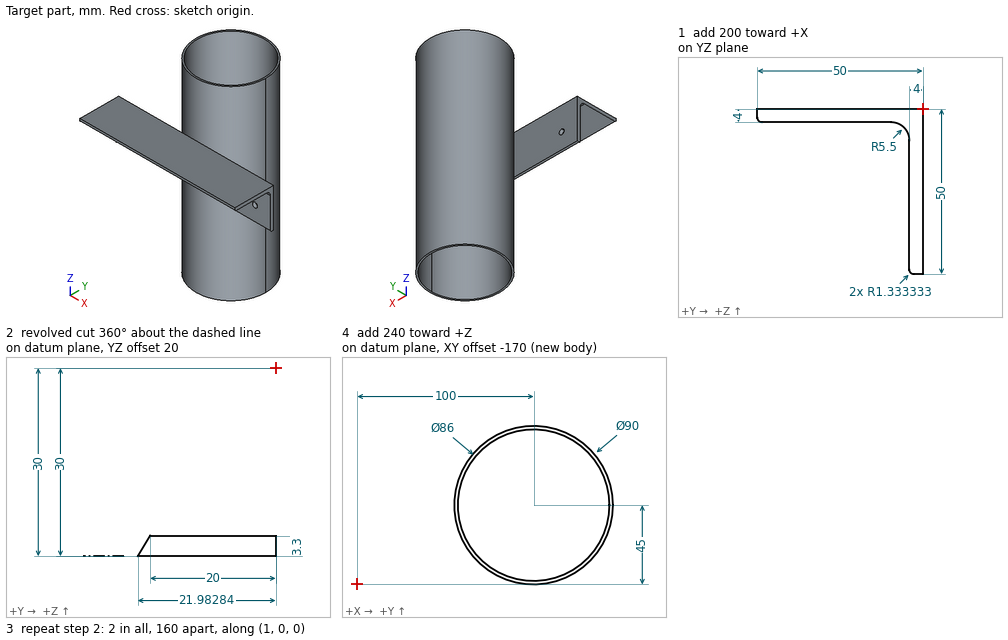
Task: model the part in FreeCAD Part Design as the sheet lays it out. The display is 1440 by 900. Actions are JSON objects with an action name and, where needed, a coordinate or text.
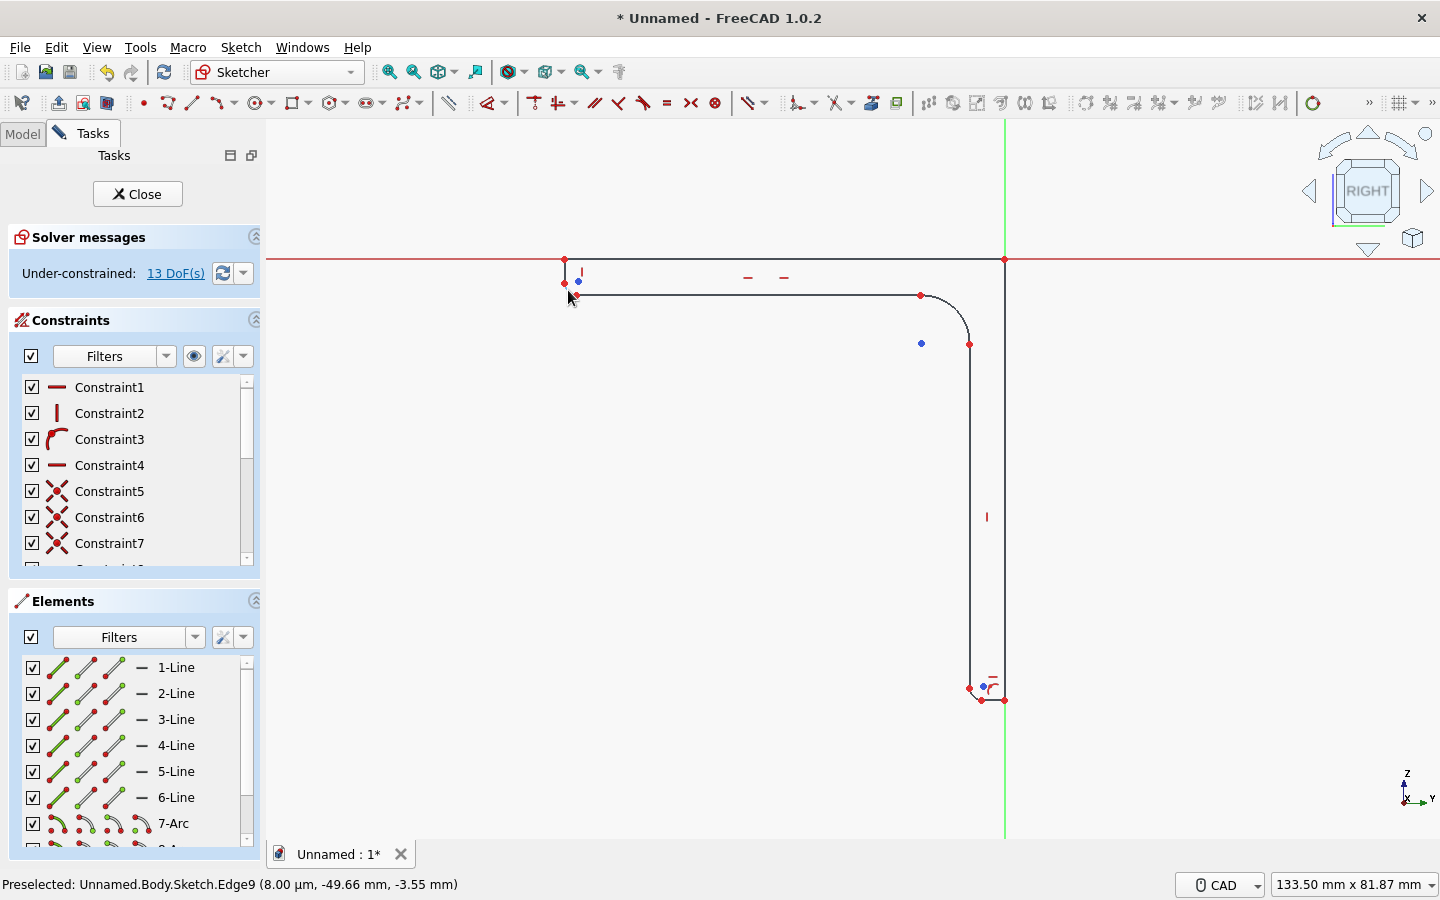
{"action": "left_click", "coordinate": [680, 295]}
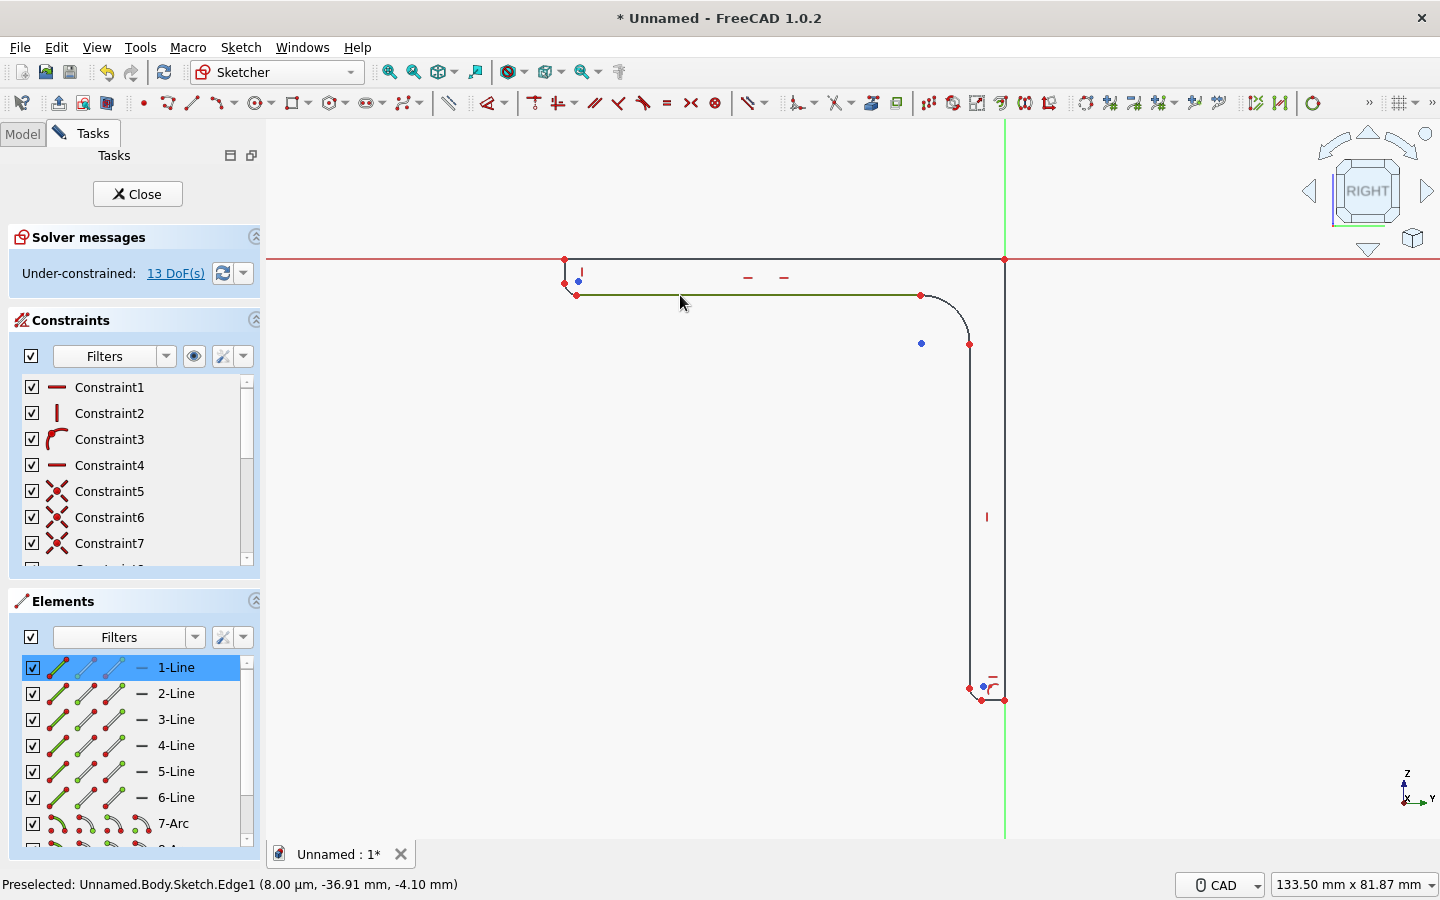
{"action": "left_click", "coordinate": [965, 322]}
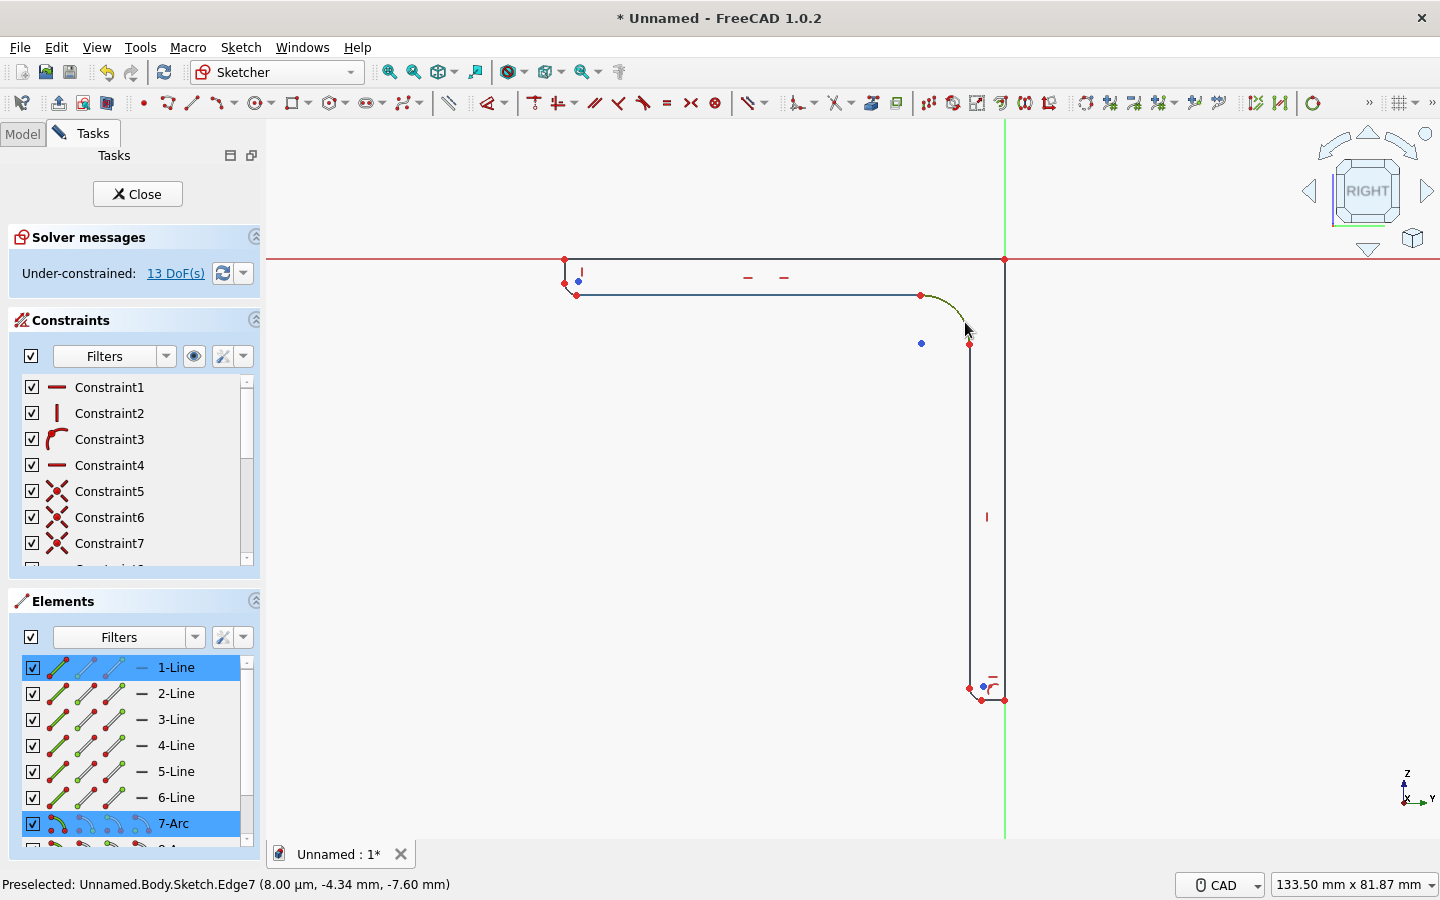
{"action": "left_click", "coordinate": [644, 104]}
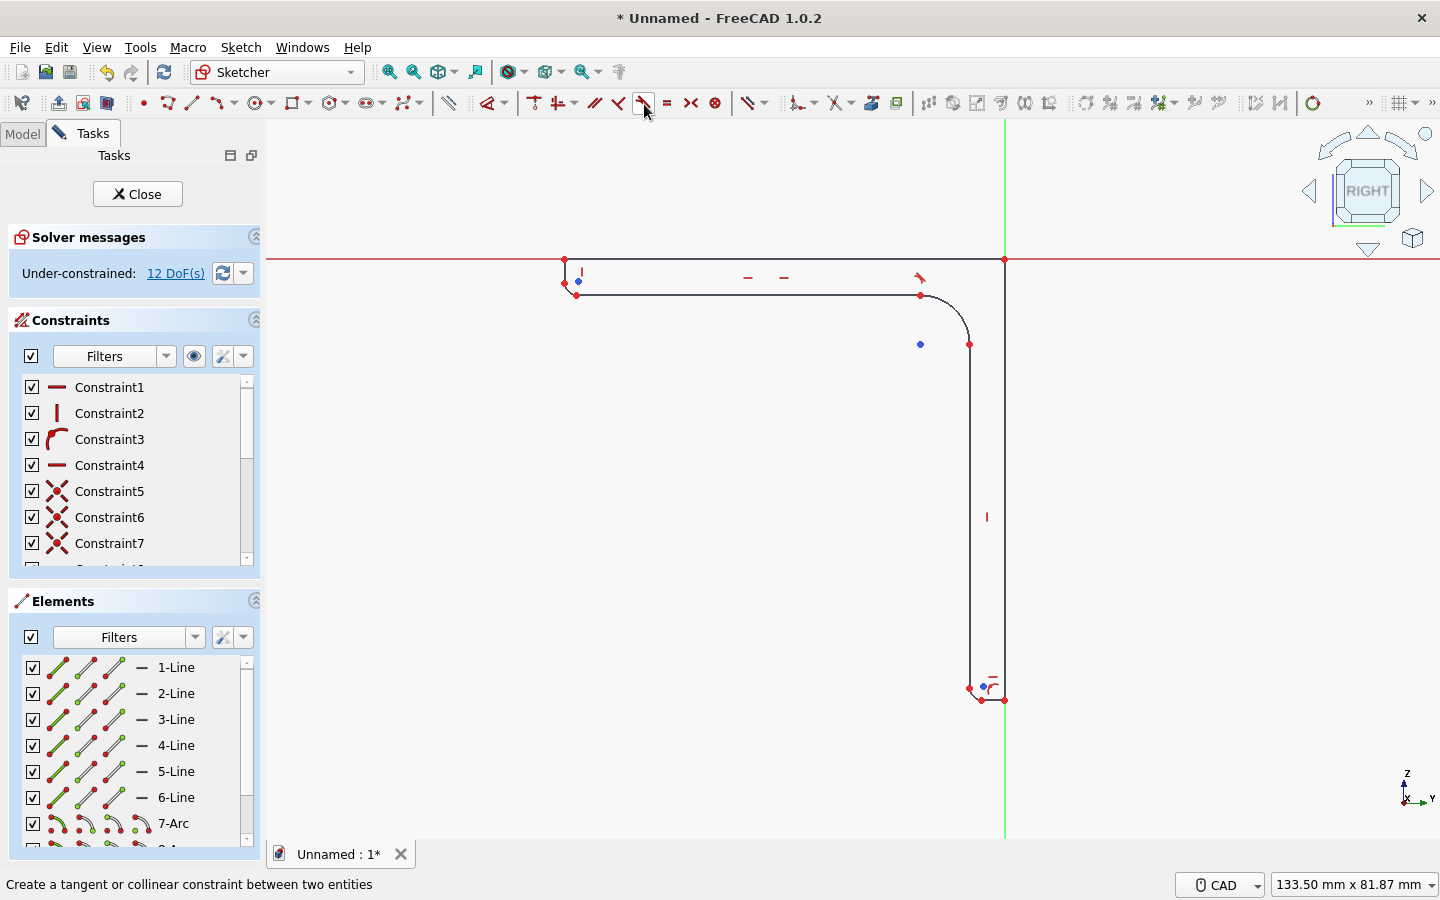
{"action": "left_click", "coordinate": [680, 295]}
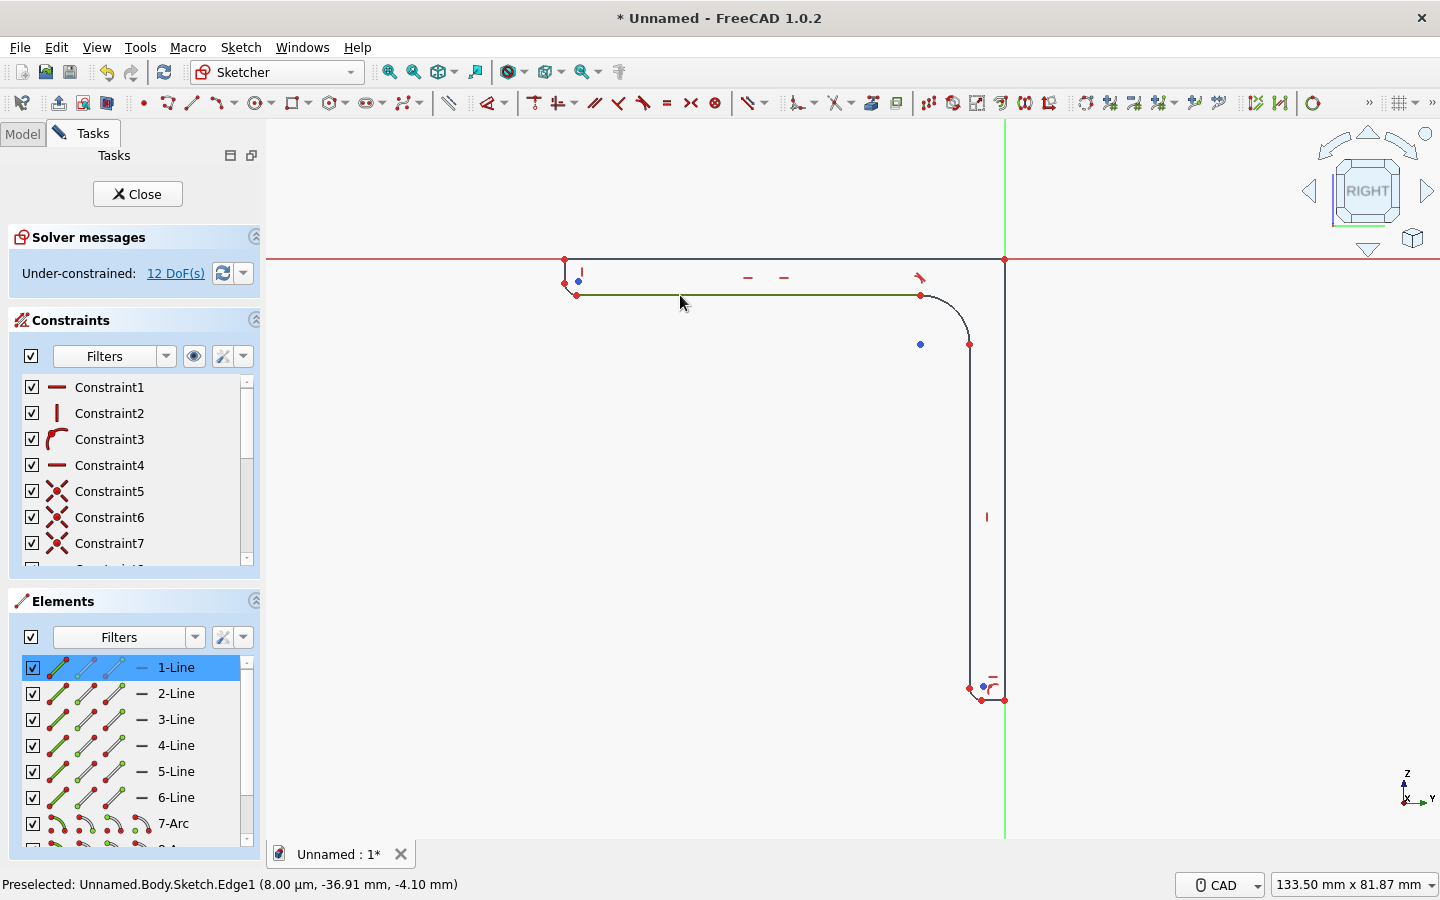
{"action": "scroll", "coordinate": [569, 291], "scroll_direction": "up", "scroll_amount": 3}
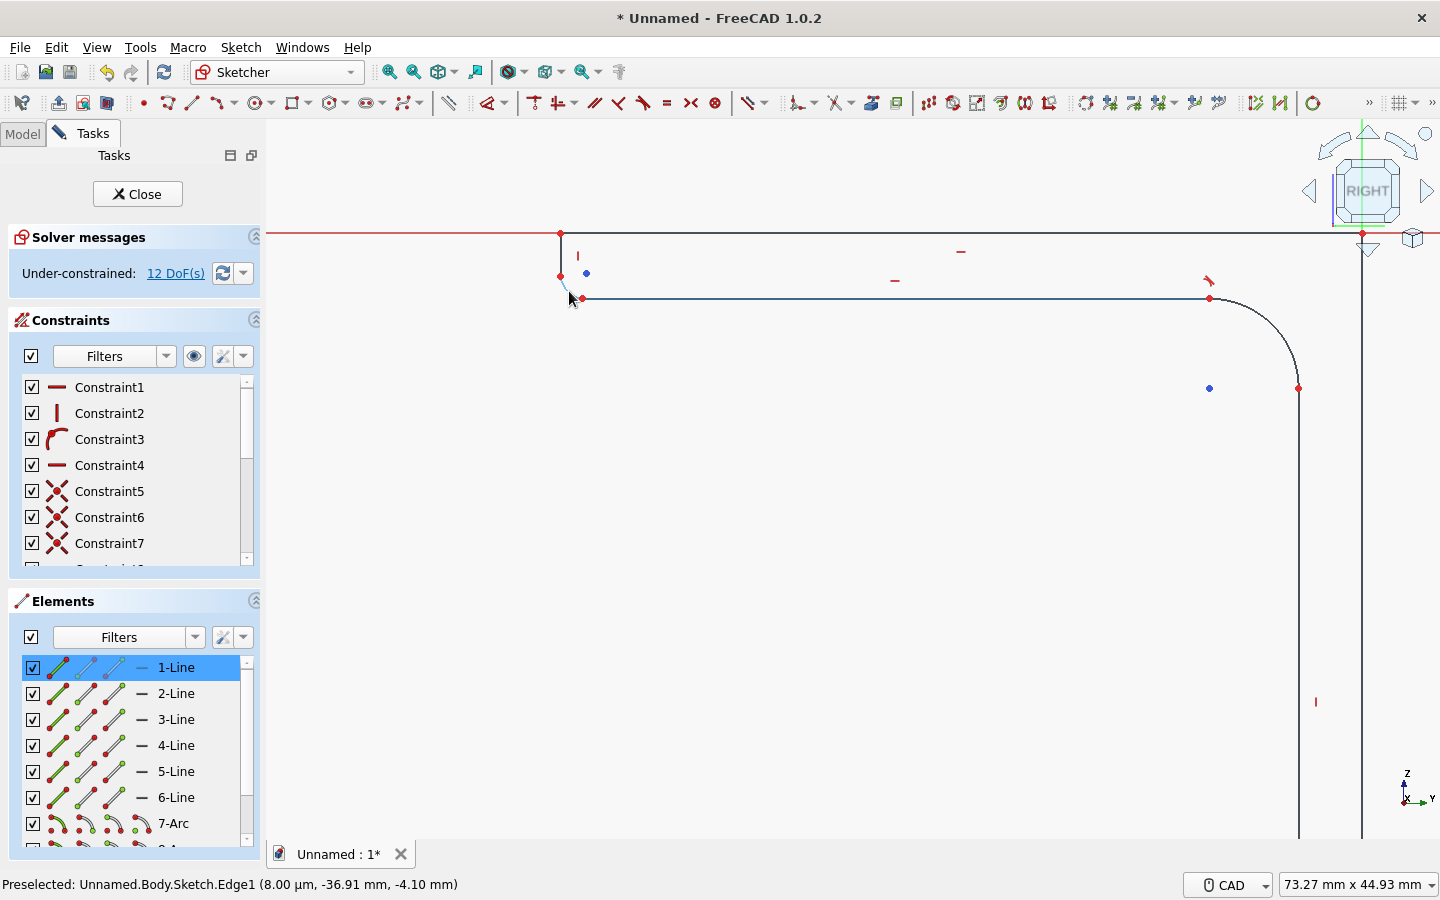
{"action": "left_click", "coordinate": [568, 291]}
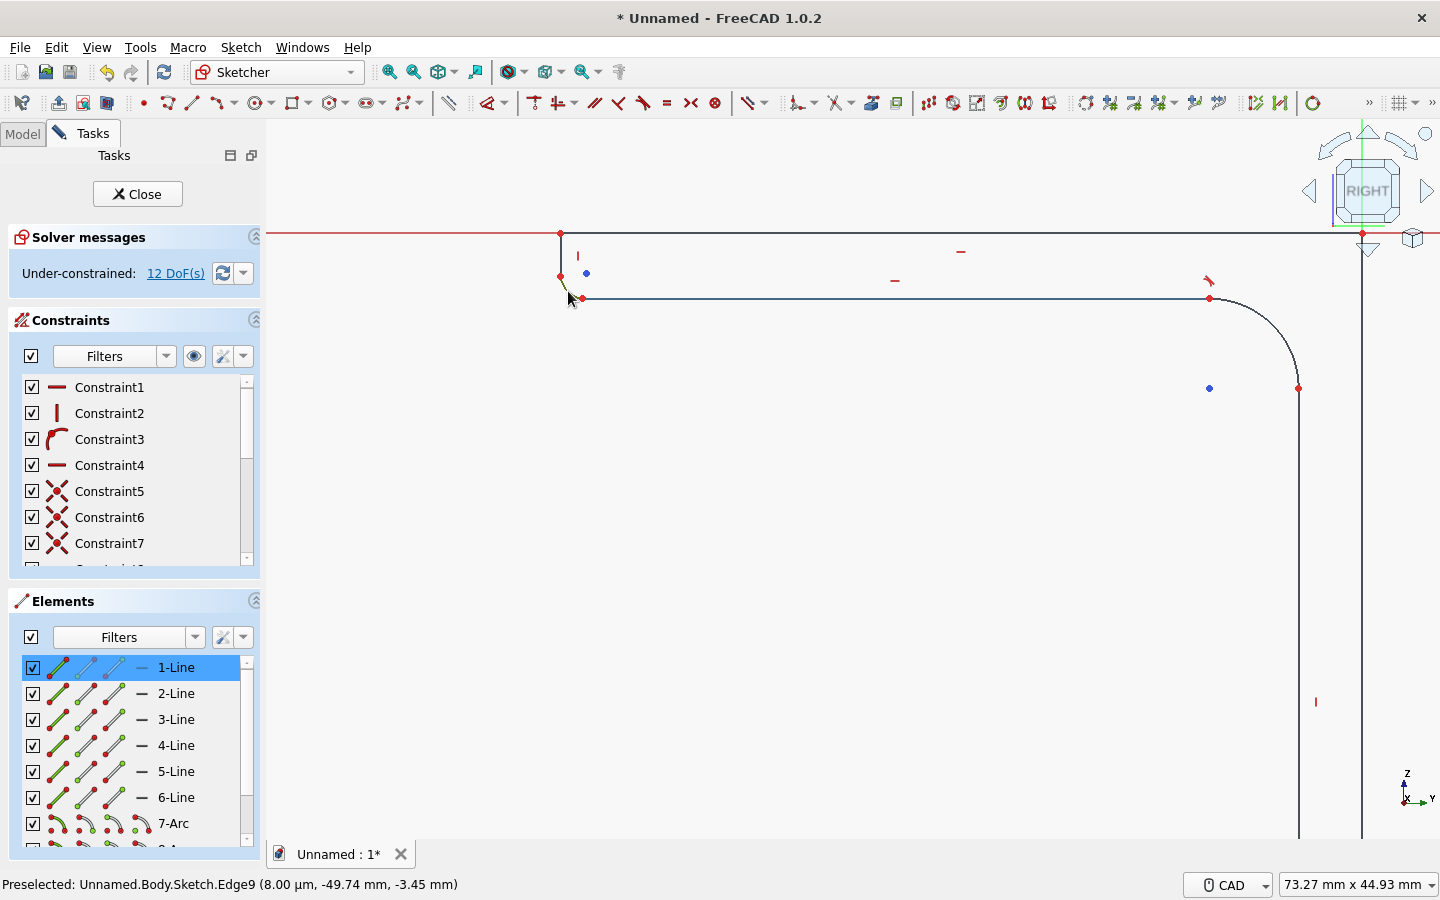
{"action": "left_click", "coordinate": [644, 104]}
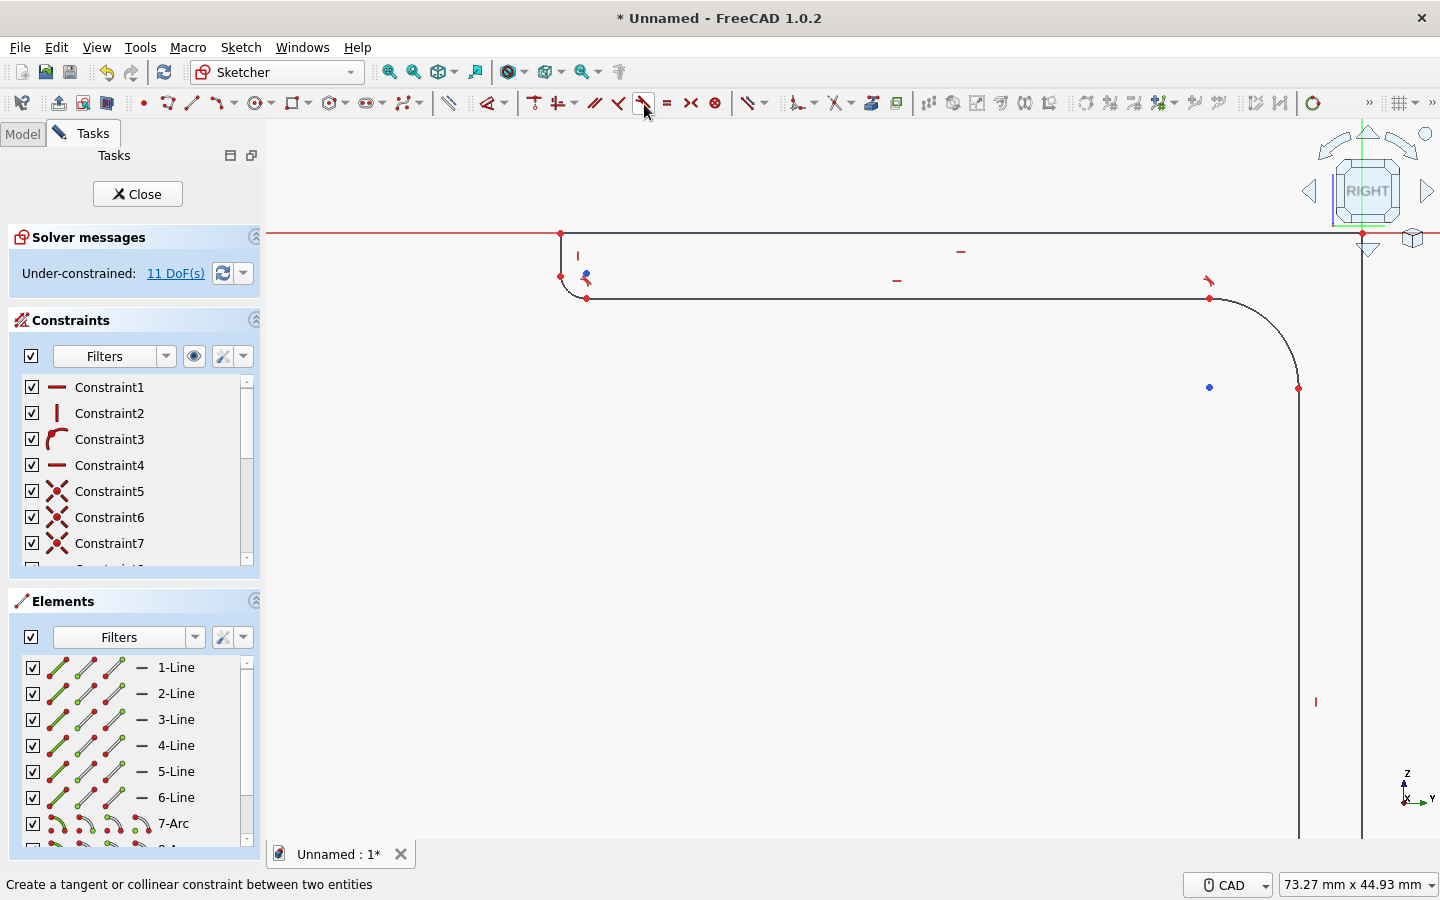
{"action": "scroll", "coordinate": [569, 291], "scroll_direction": "down", "scroll_amount": 3}